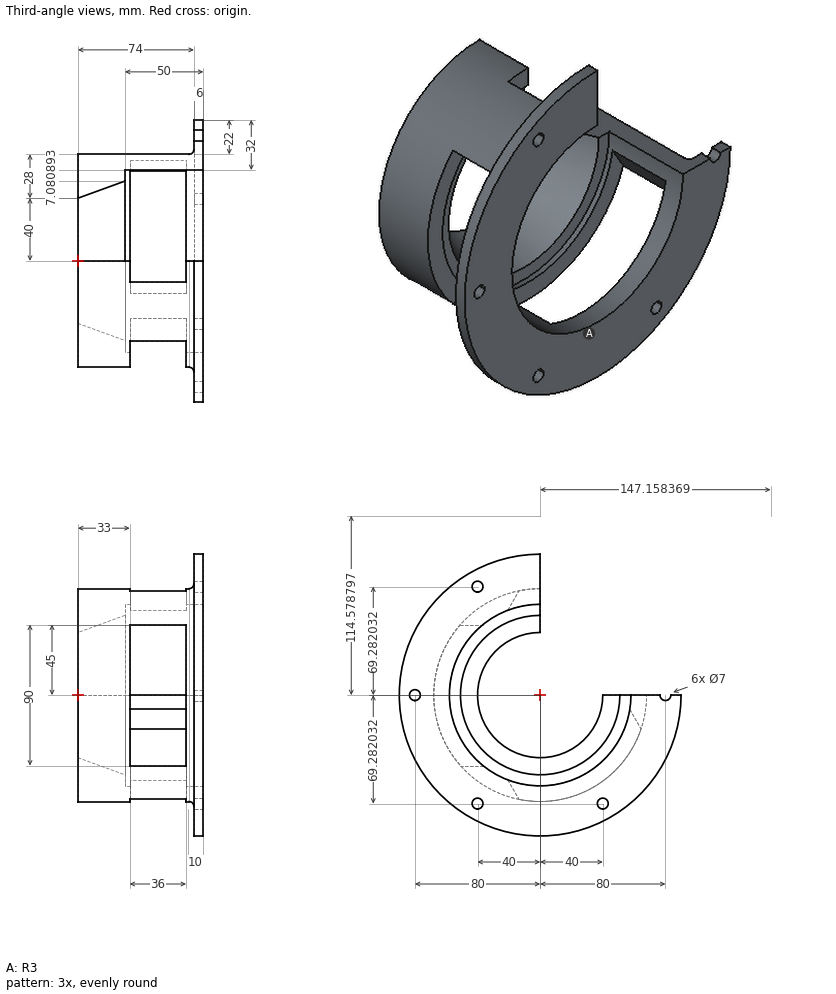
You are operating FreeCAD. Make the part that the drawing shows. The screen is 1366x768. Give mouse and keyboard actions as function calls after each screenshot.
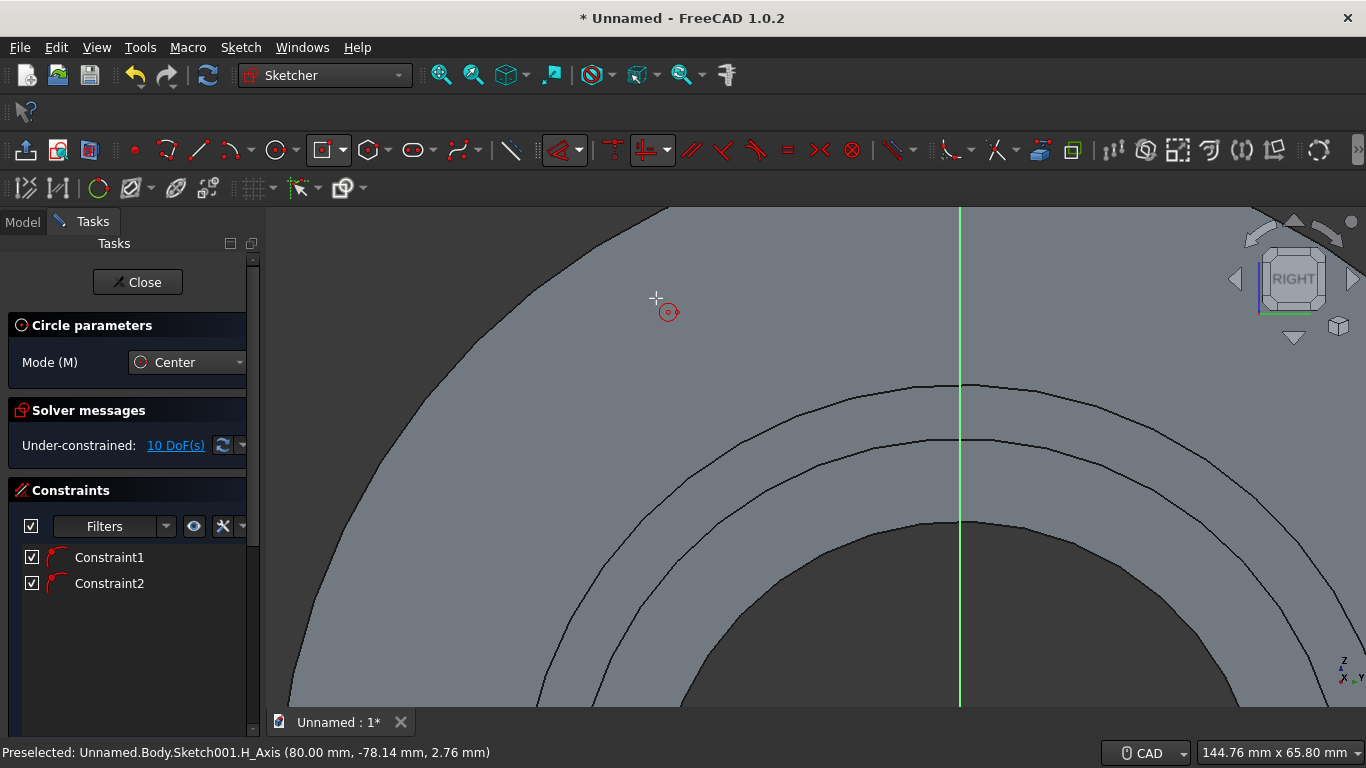
scroll(656, 298, down, 6)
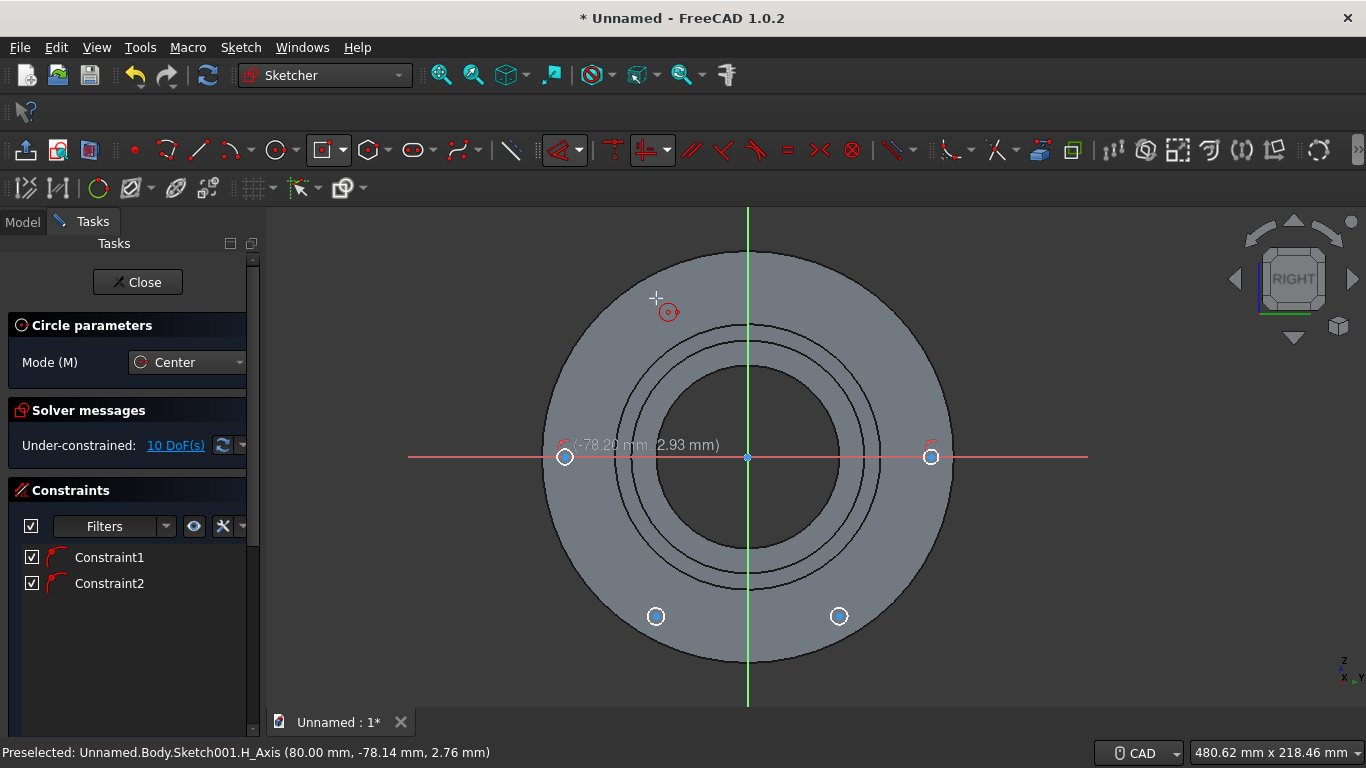
click(656, 298)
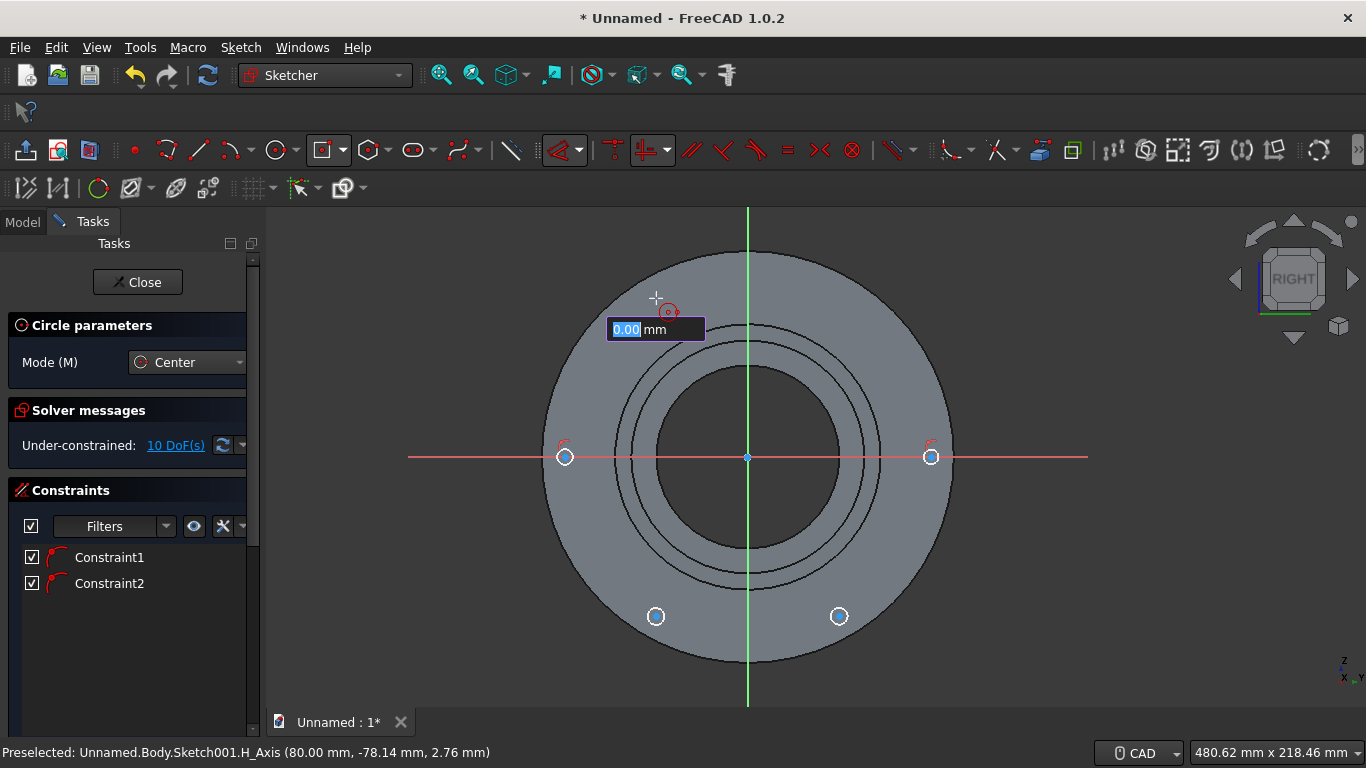
scroll(662, 293, up, 4)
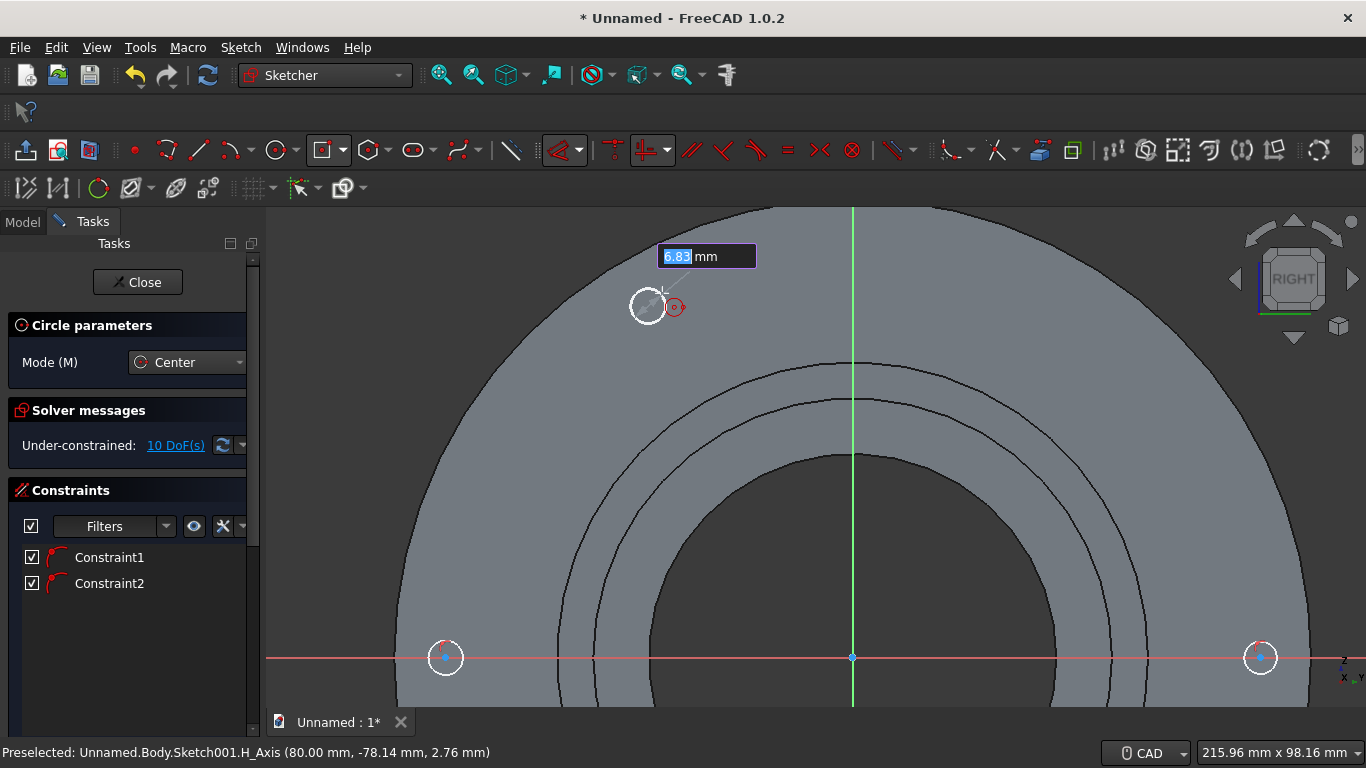
click(661, 292)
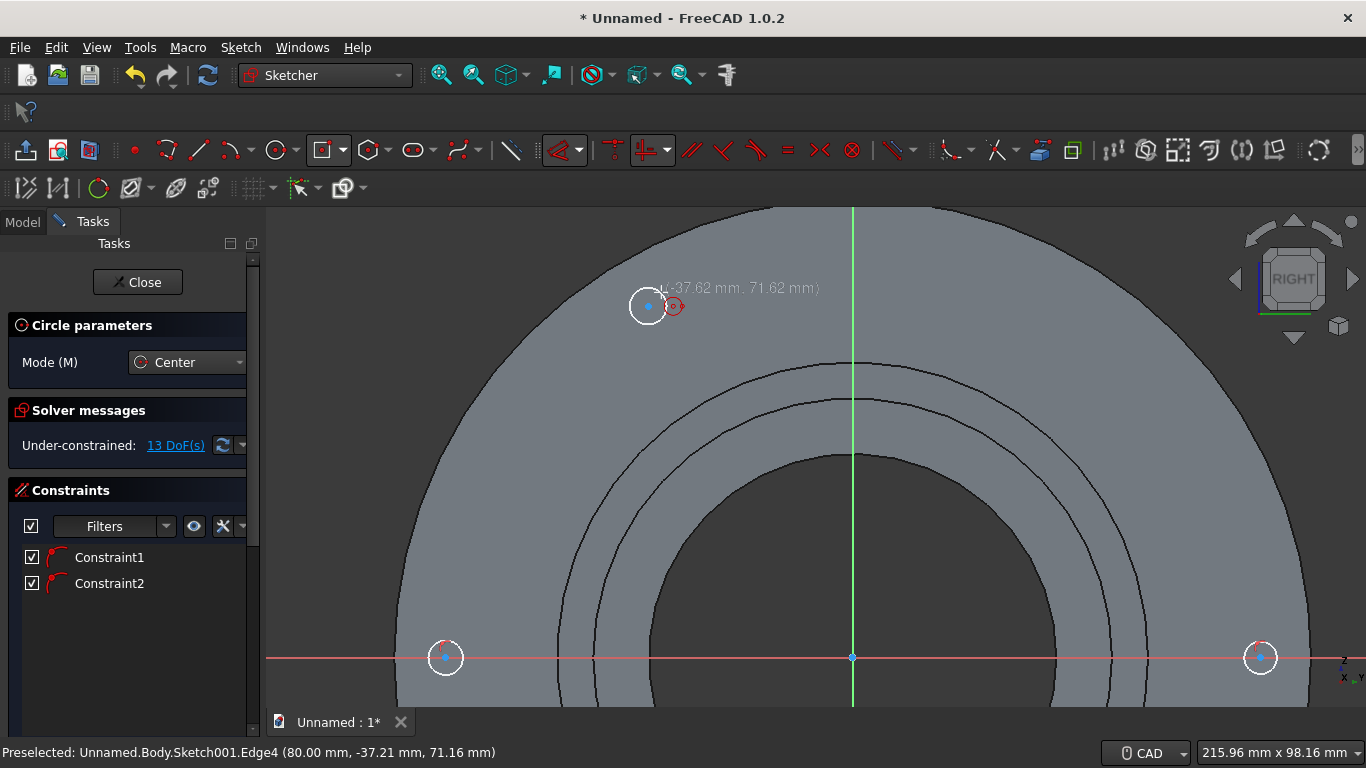
scroll(1056, 305, up, 2)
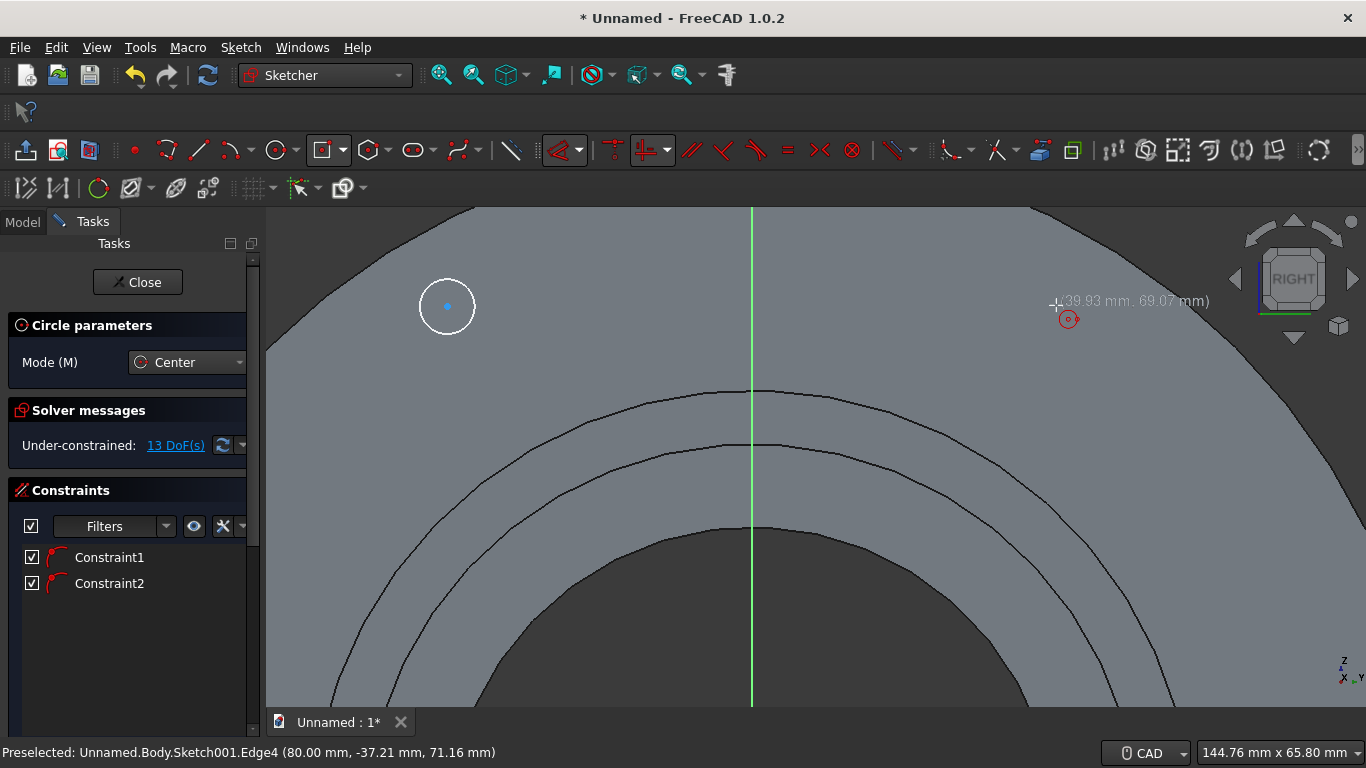
scroll(745, 296, down, 6)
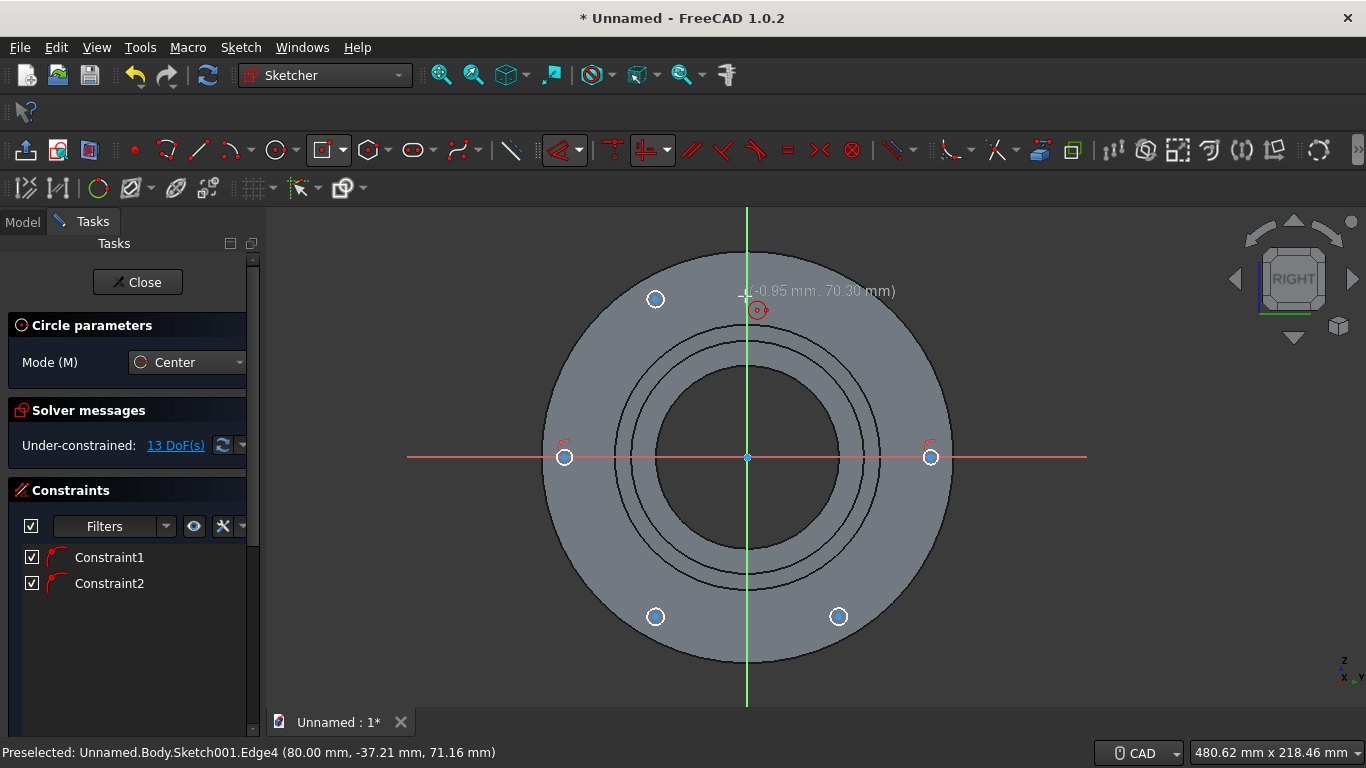
click(839, 299)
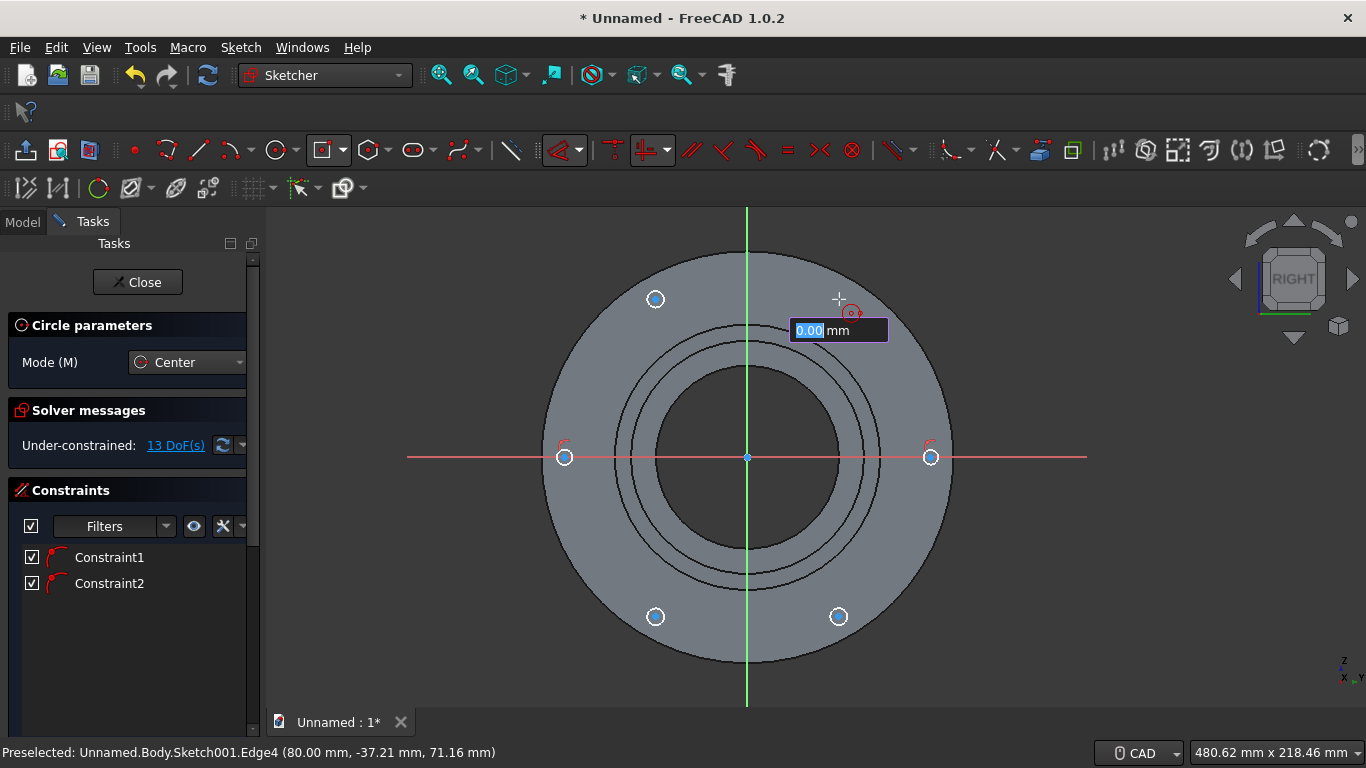
scroll(845, 293, up, 4)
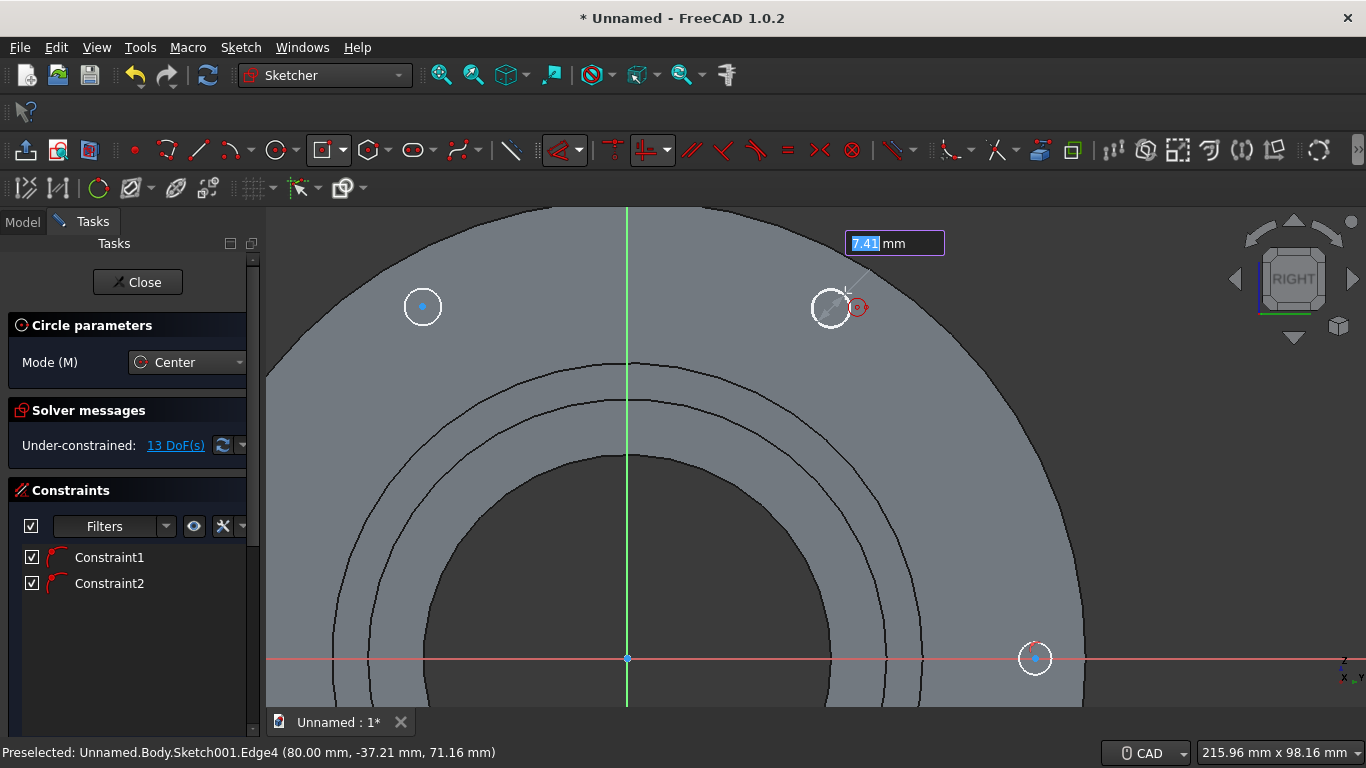
click(844, 293)
key(Escape)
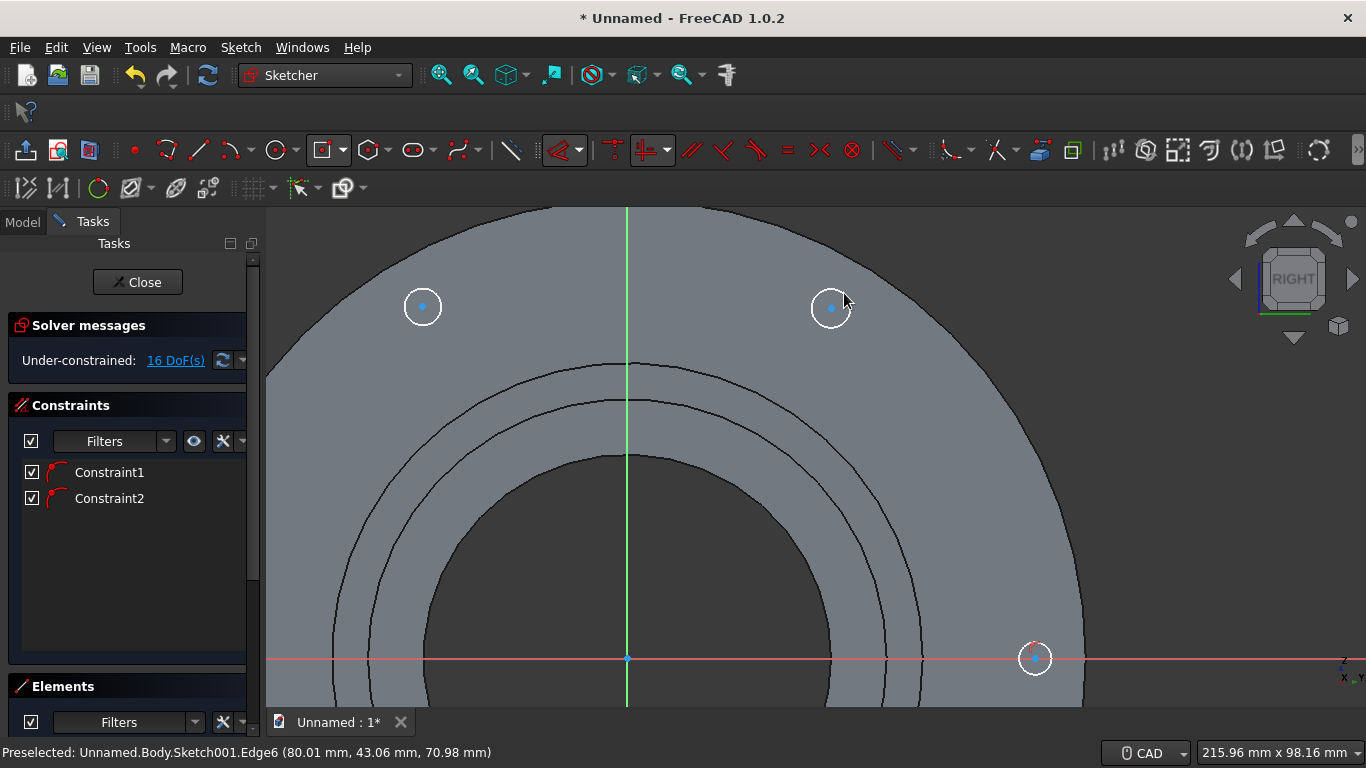
click(1047, 647)